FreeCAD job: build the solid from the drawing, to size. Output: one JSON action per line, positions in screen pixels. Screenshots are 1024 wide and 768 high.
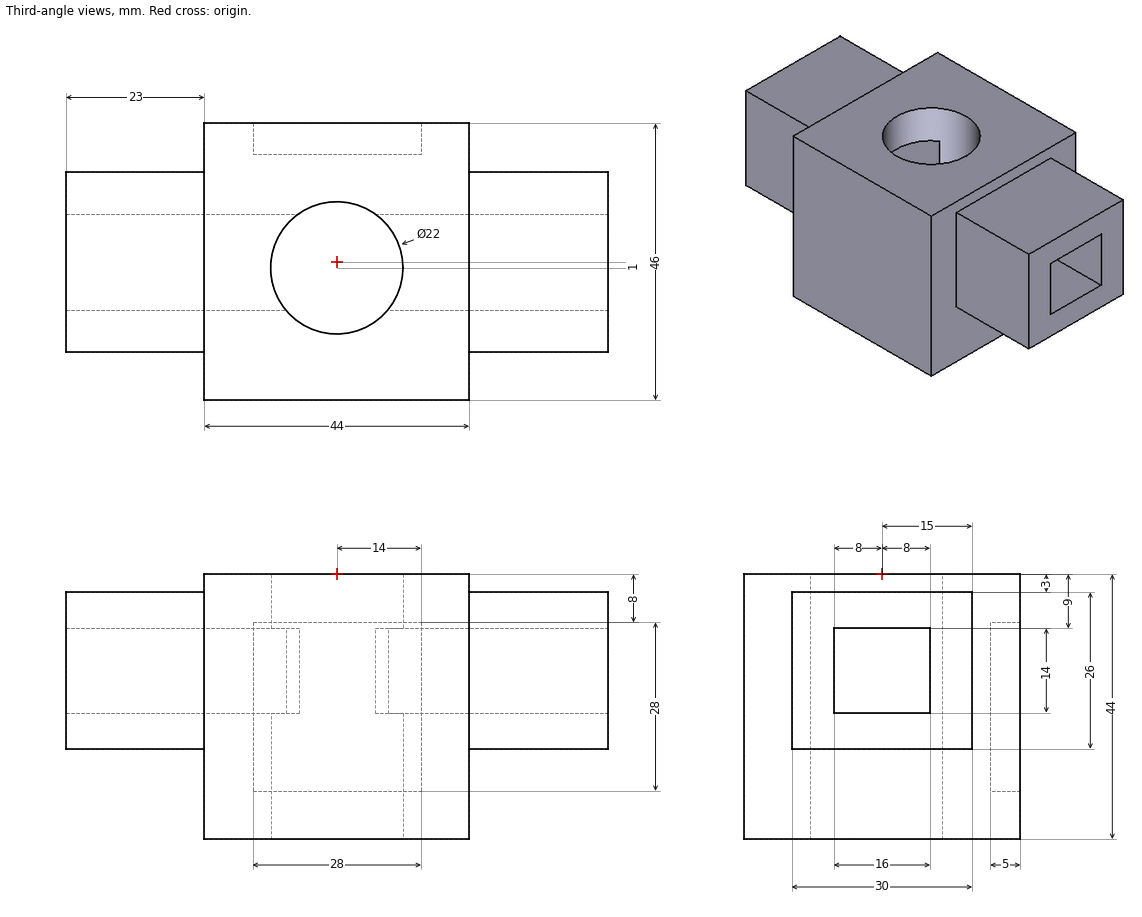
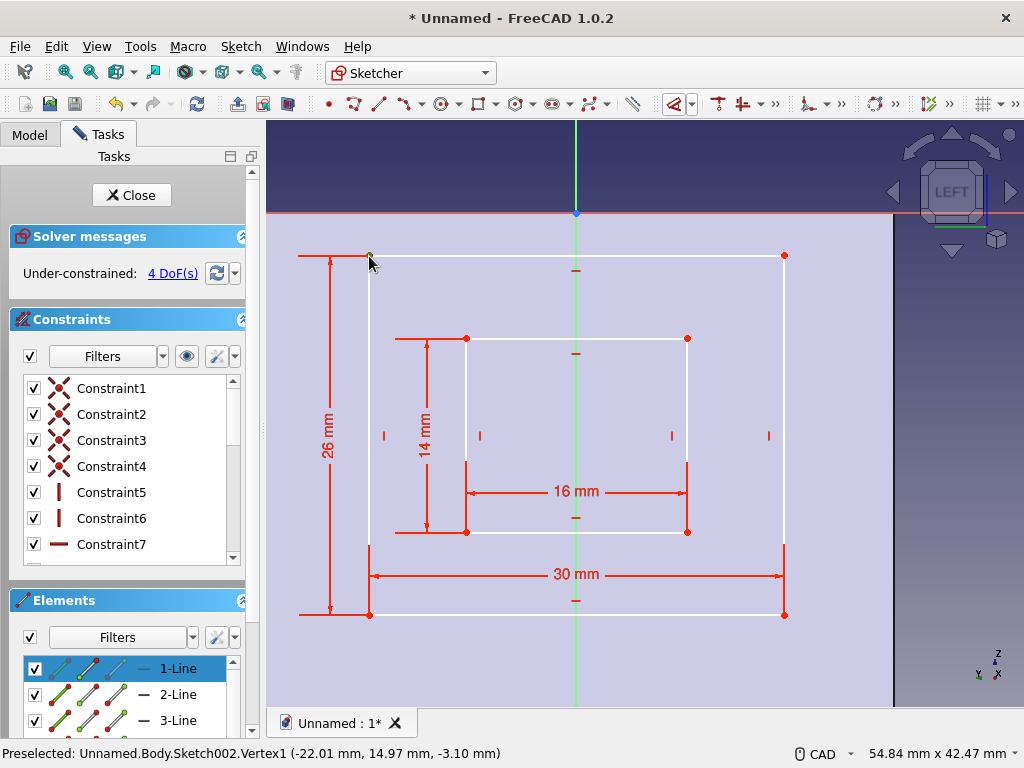
{"action": "key", "text": "i"}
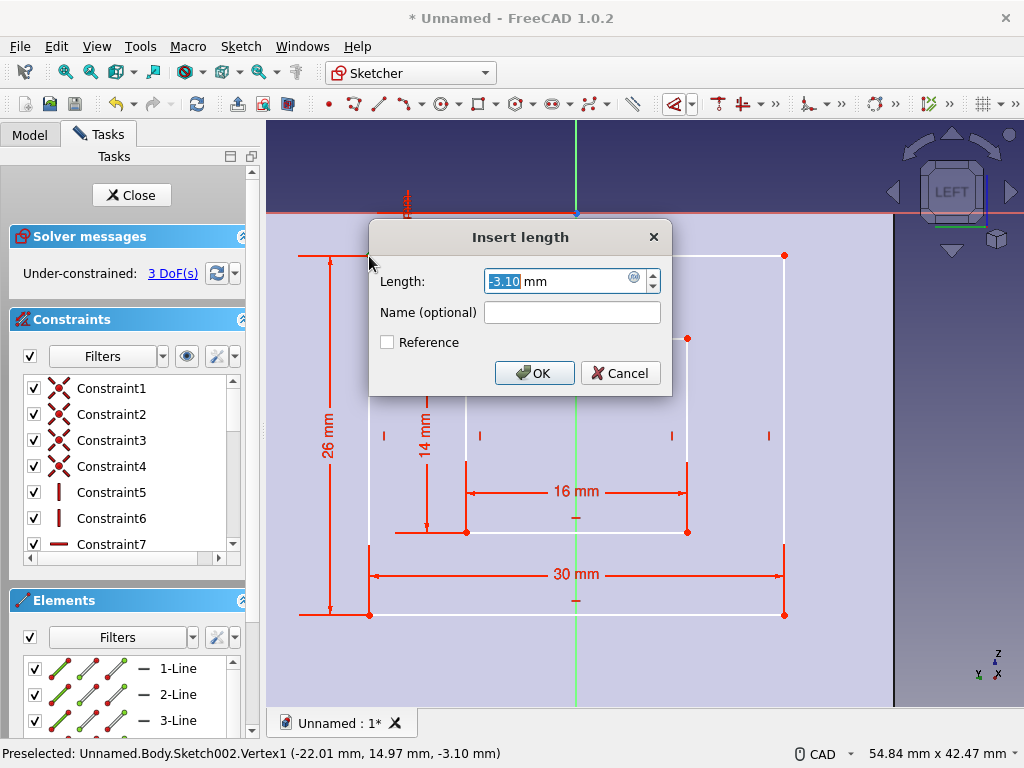
{"action": "type", "text": "-3"}
{"action": "key", "text": "Return"}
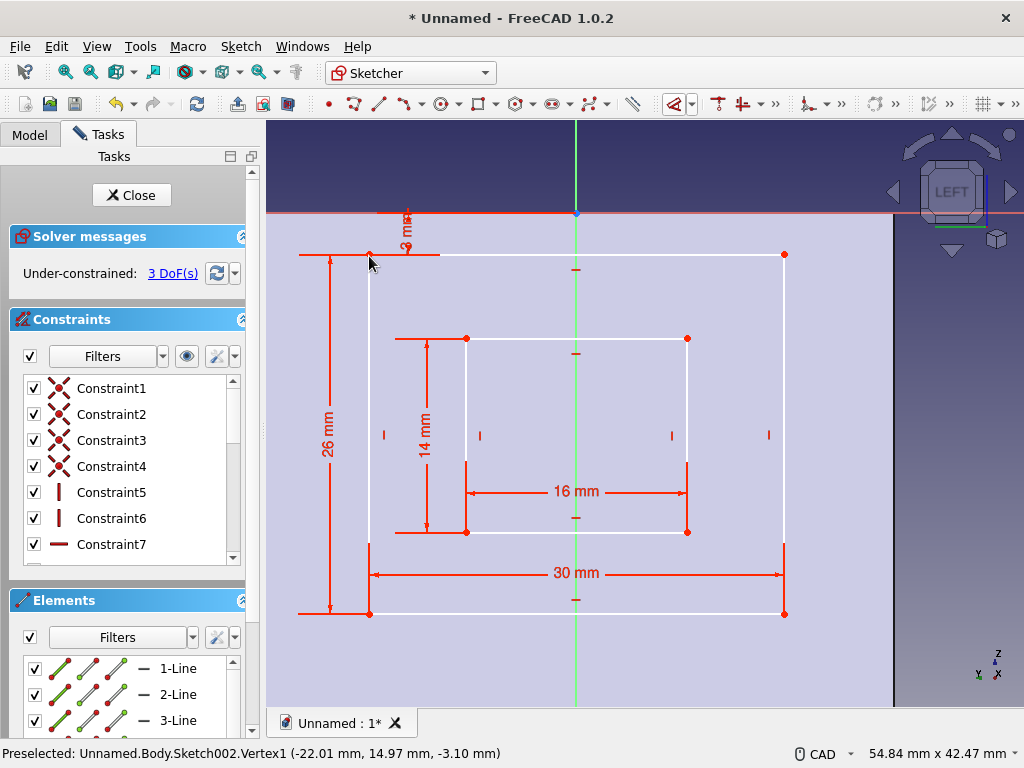
{"action": "left_click", "coordinate": [466, 339]}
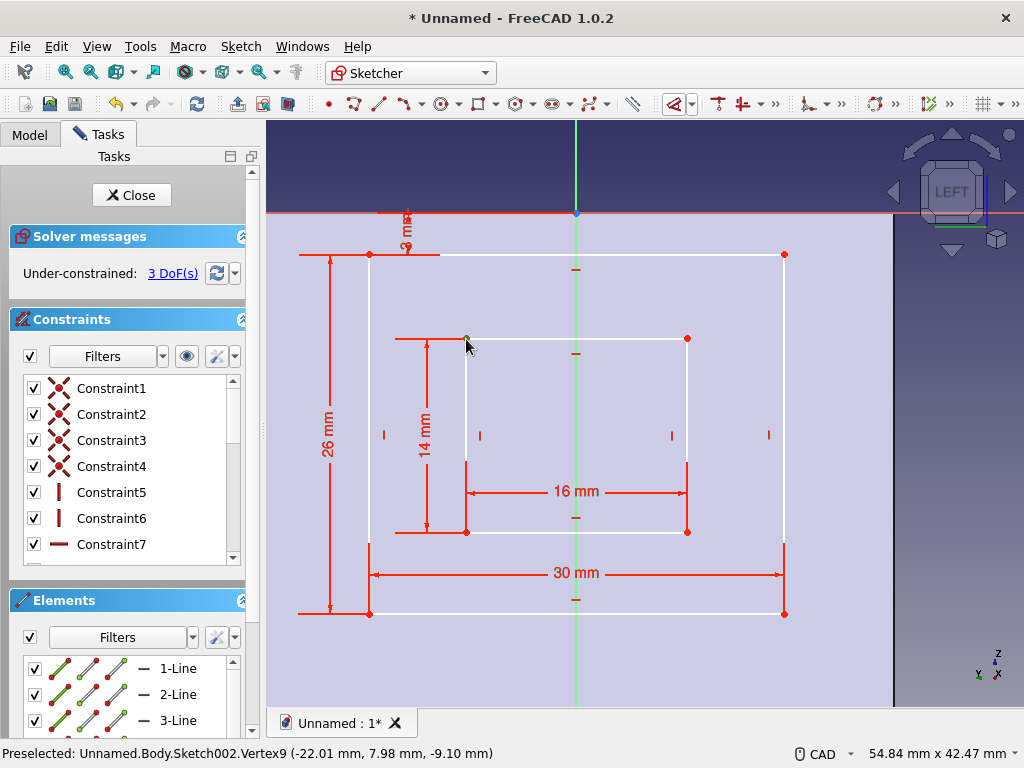
{"action": "key", "text": "l"}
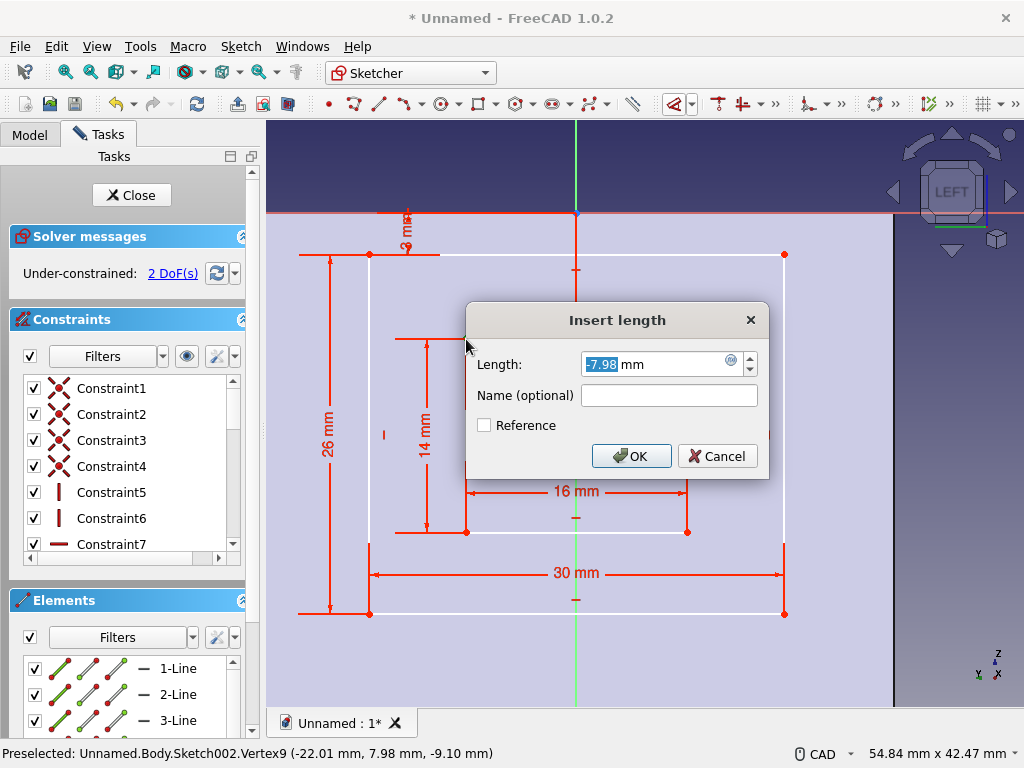
{"action": "type", "text": "-8"}
{"action": "key", "text": "Return"}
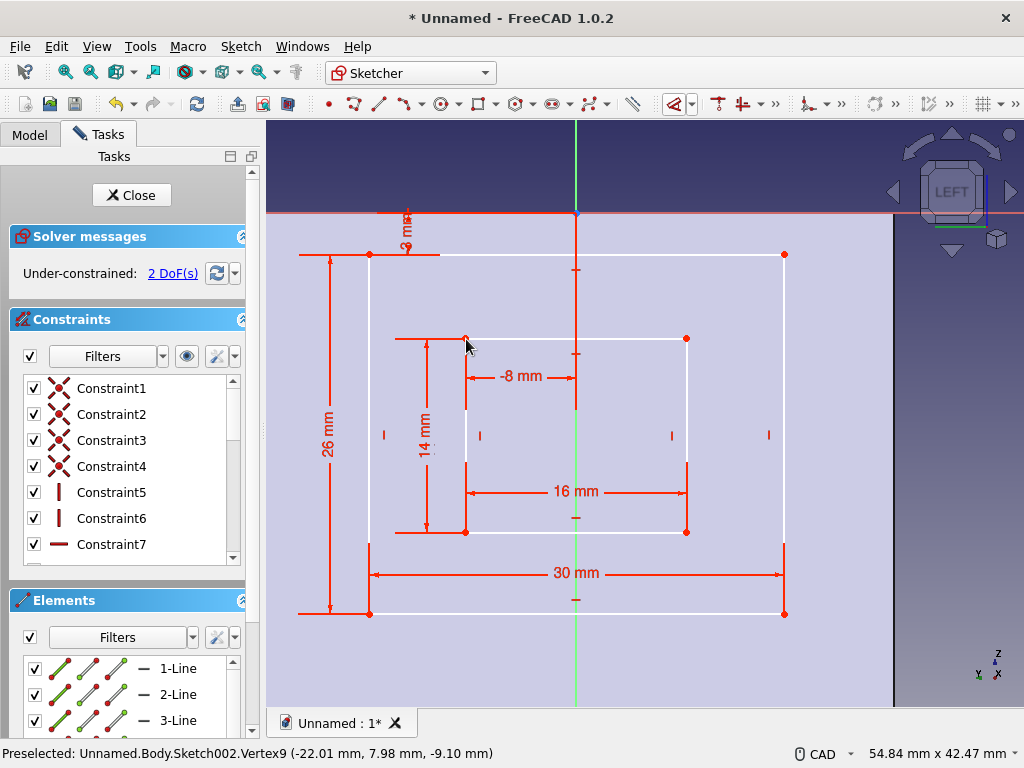
{"action": "left_click", "coordinate": [466, 339]}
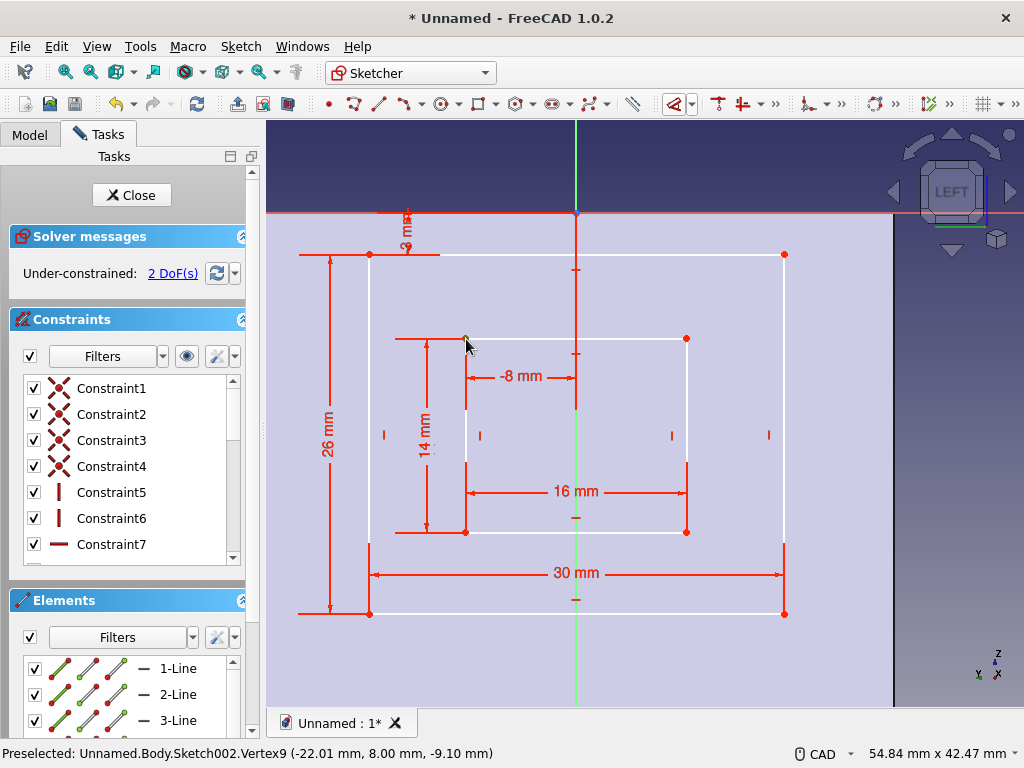
{"action": "key", "text": "i"}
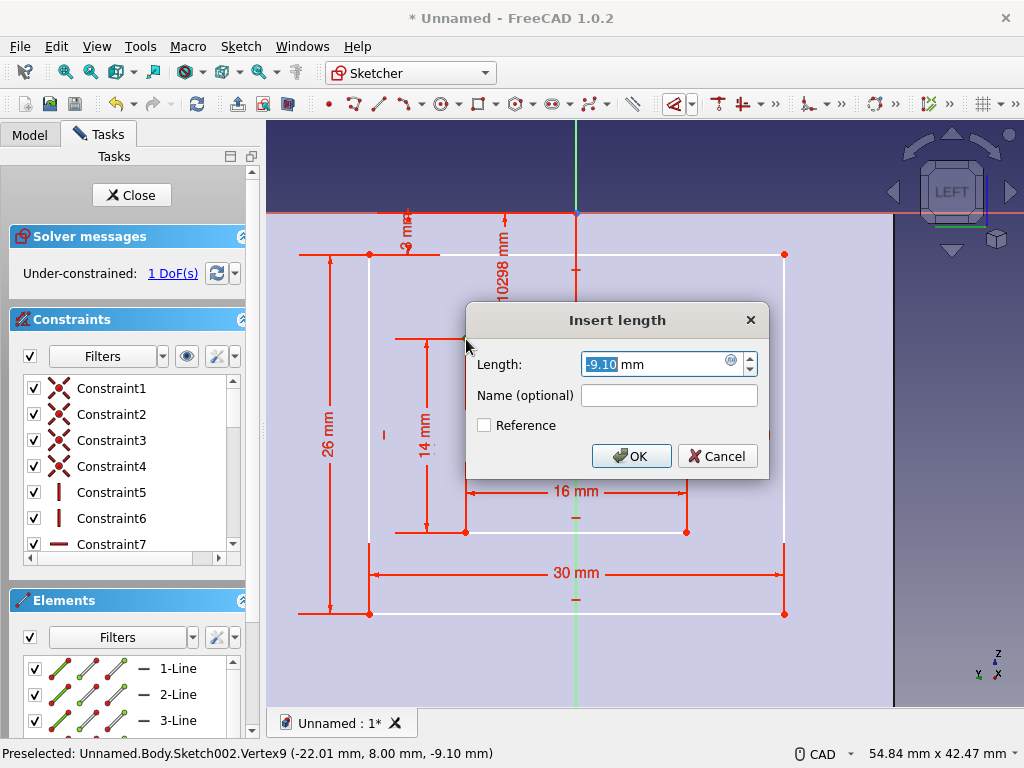
{"action": "type", "text": "-9"}
{"action": "key", "text": "Return"}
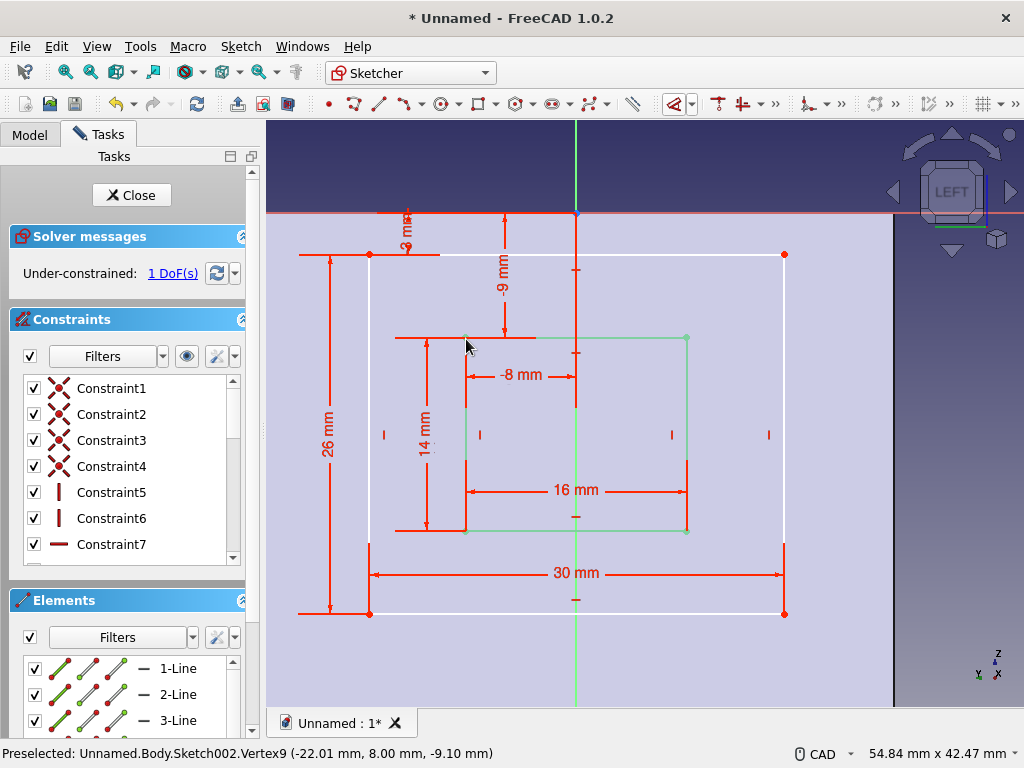
{"action": "left_click", "coordinate": [369, 255]}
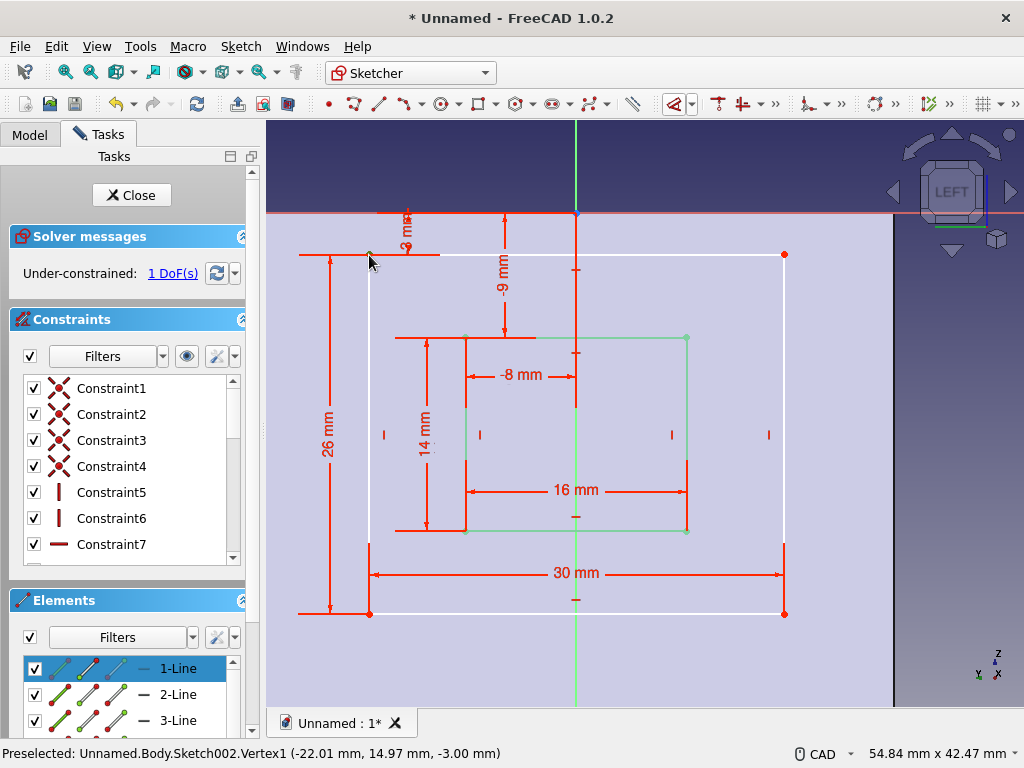
{"action": "key", "text": "l"}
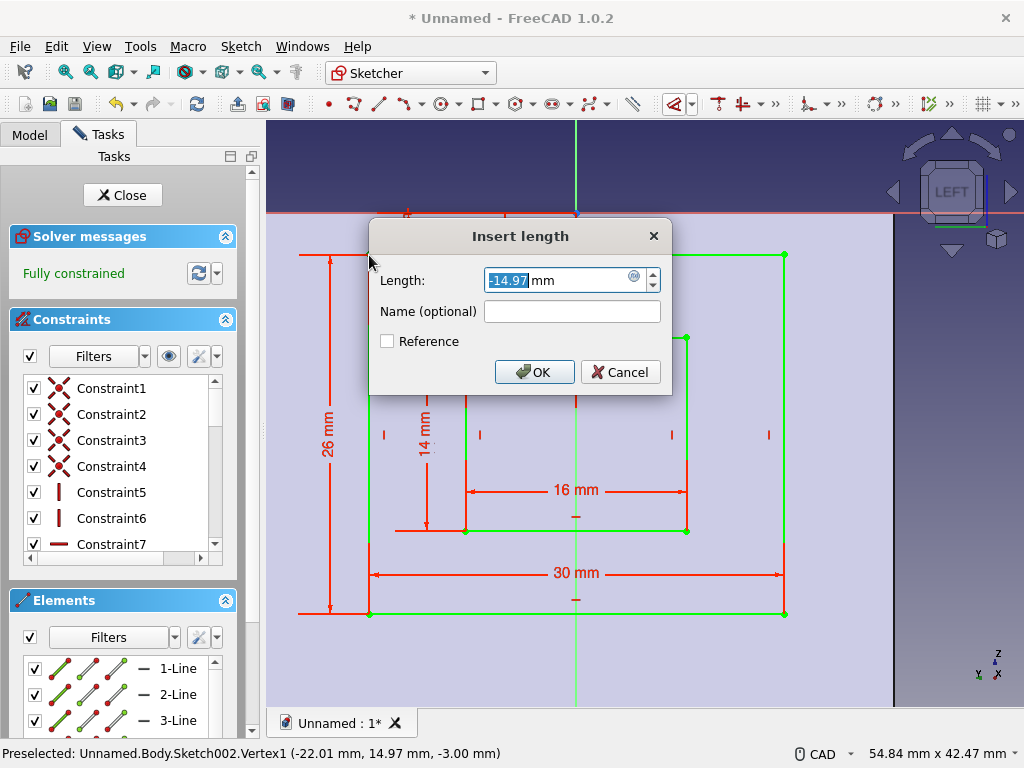
{"action": "type", "text": "-15"}
{"action": "key", "text": "Return"}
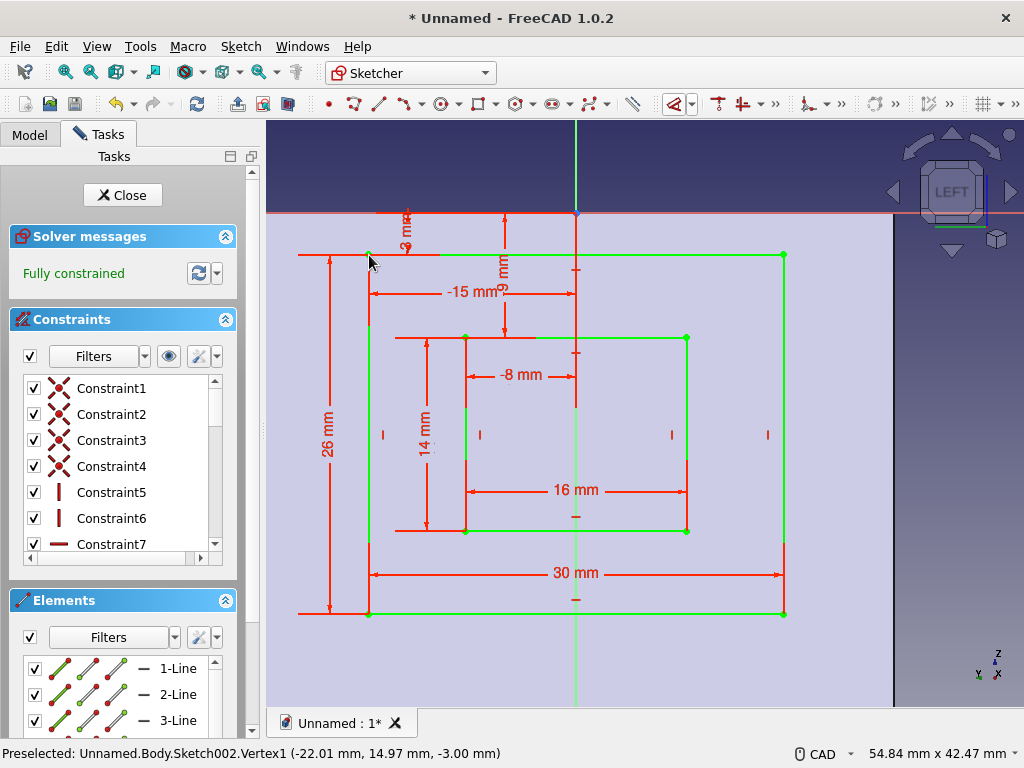
{"action": "left_click", "coordinate": [123, 195]}